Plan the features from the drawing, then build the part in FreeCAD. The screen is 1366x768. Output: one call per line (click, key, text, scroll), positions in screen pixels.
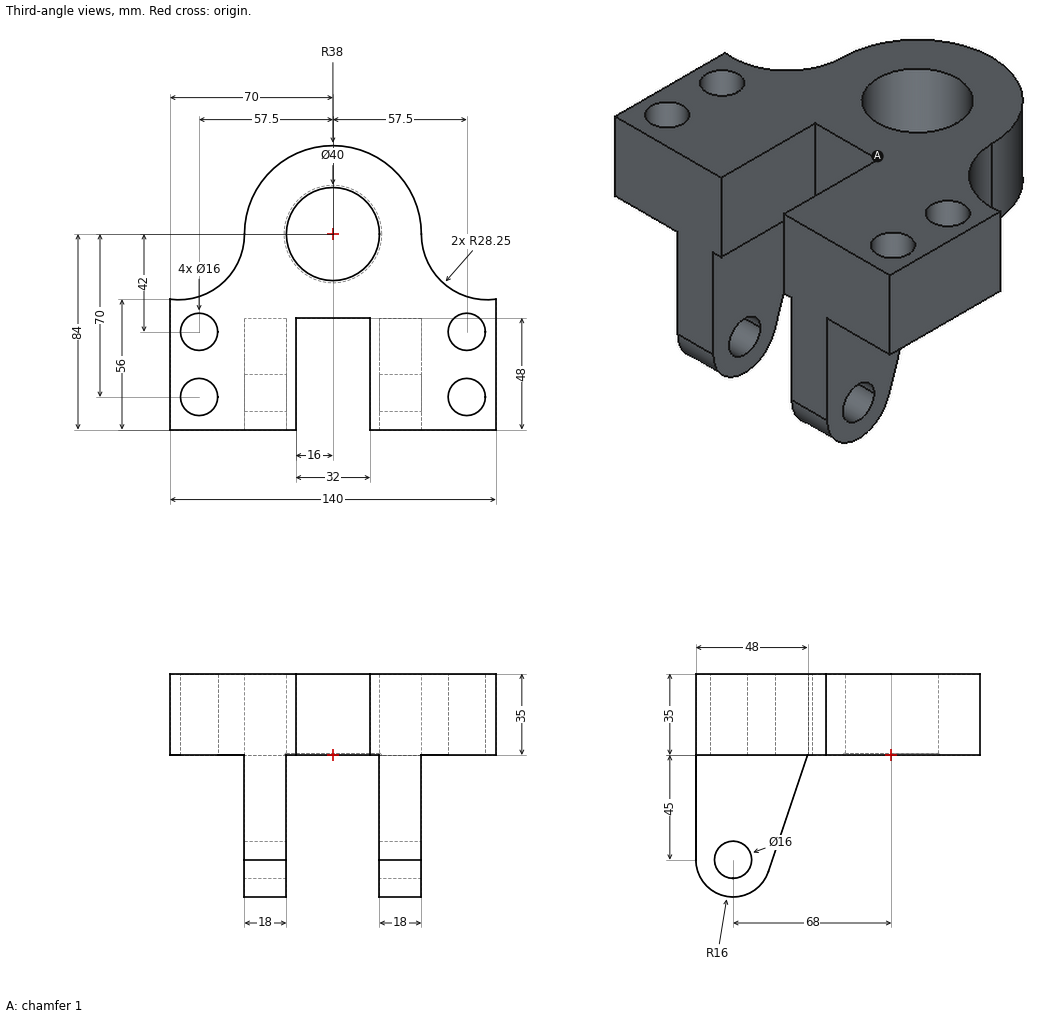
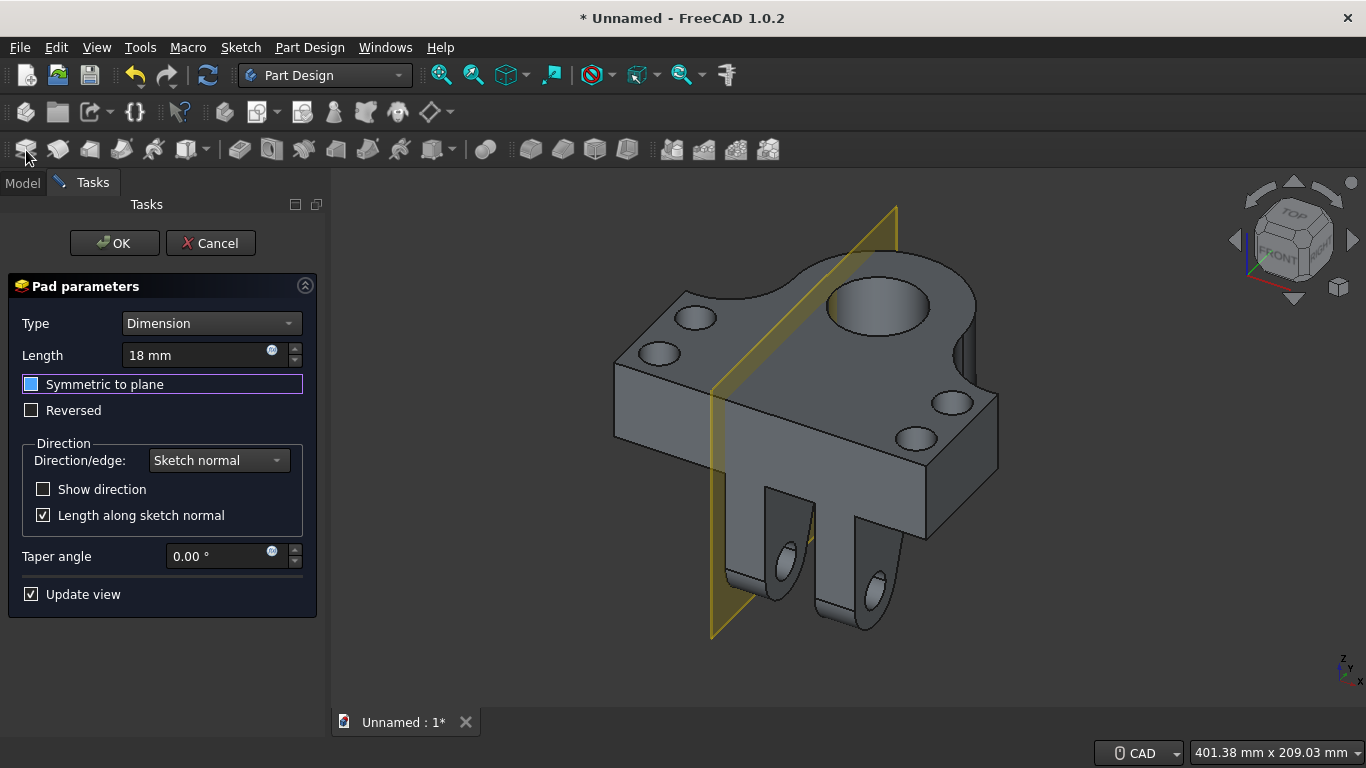
click(30, 410)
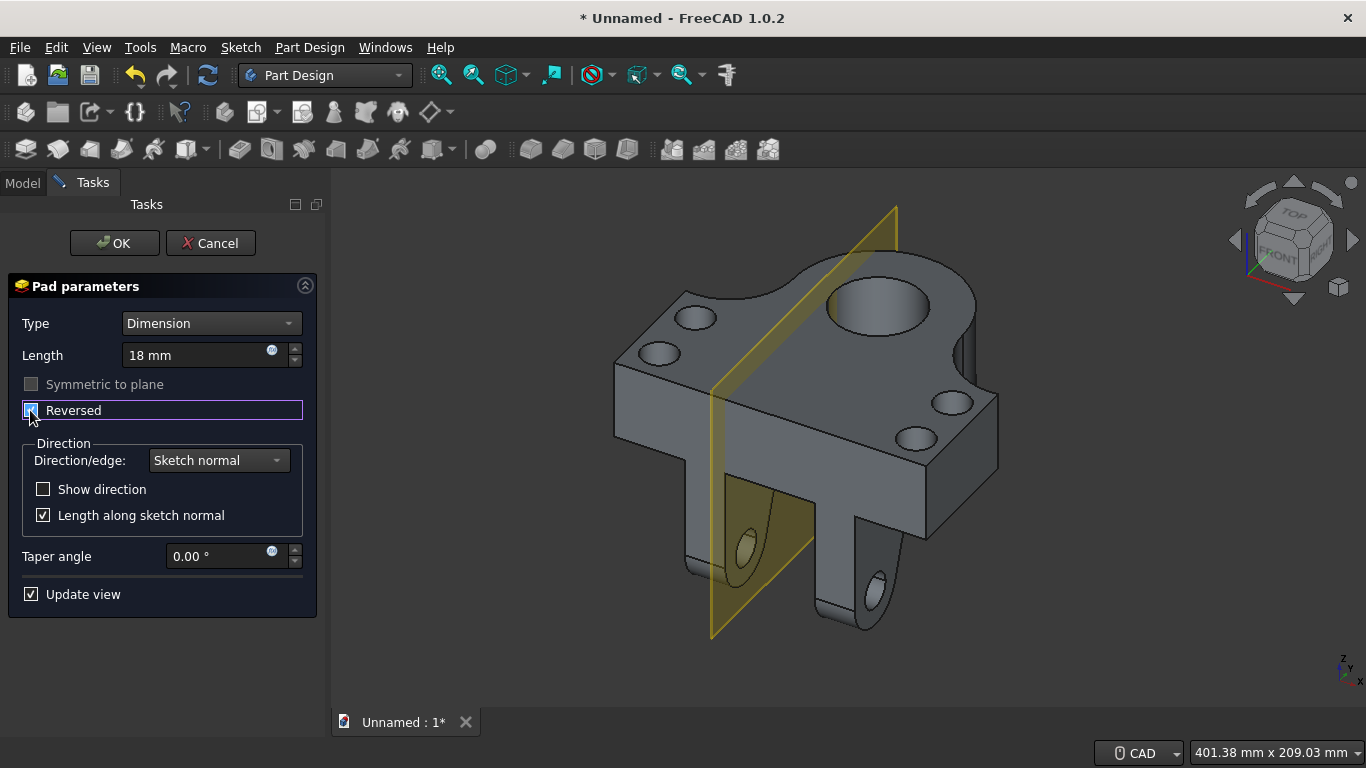
click(115, 243)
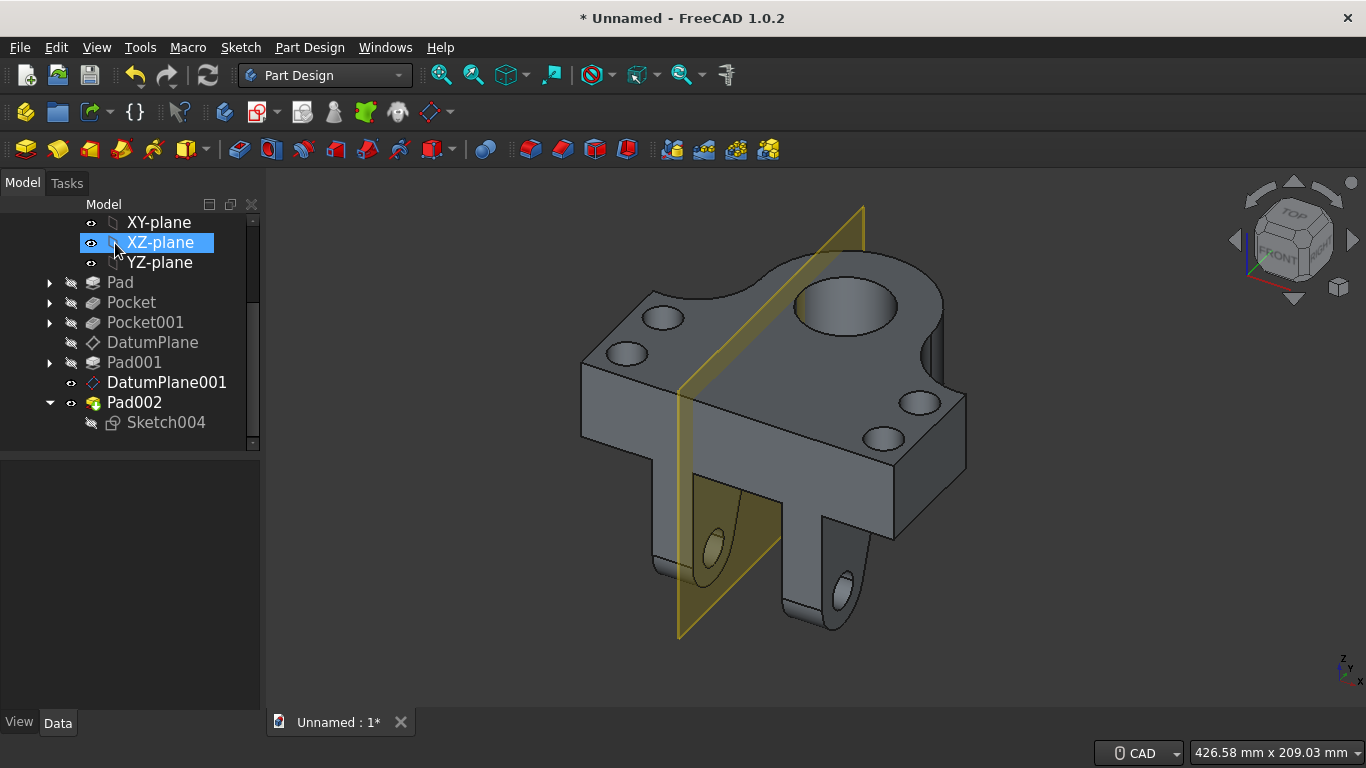
click(116, 383)
key(space)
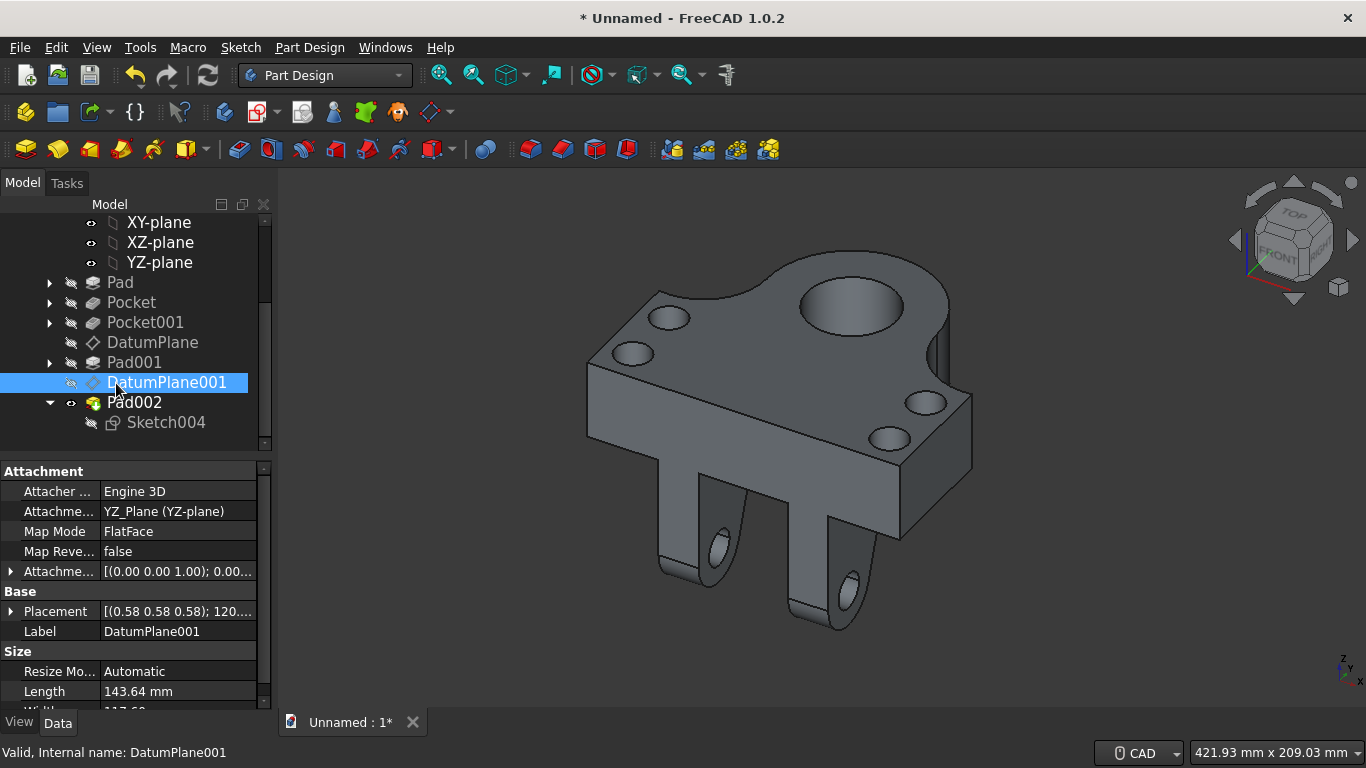
key(5)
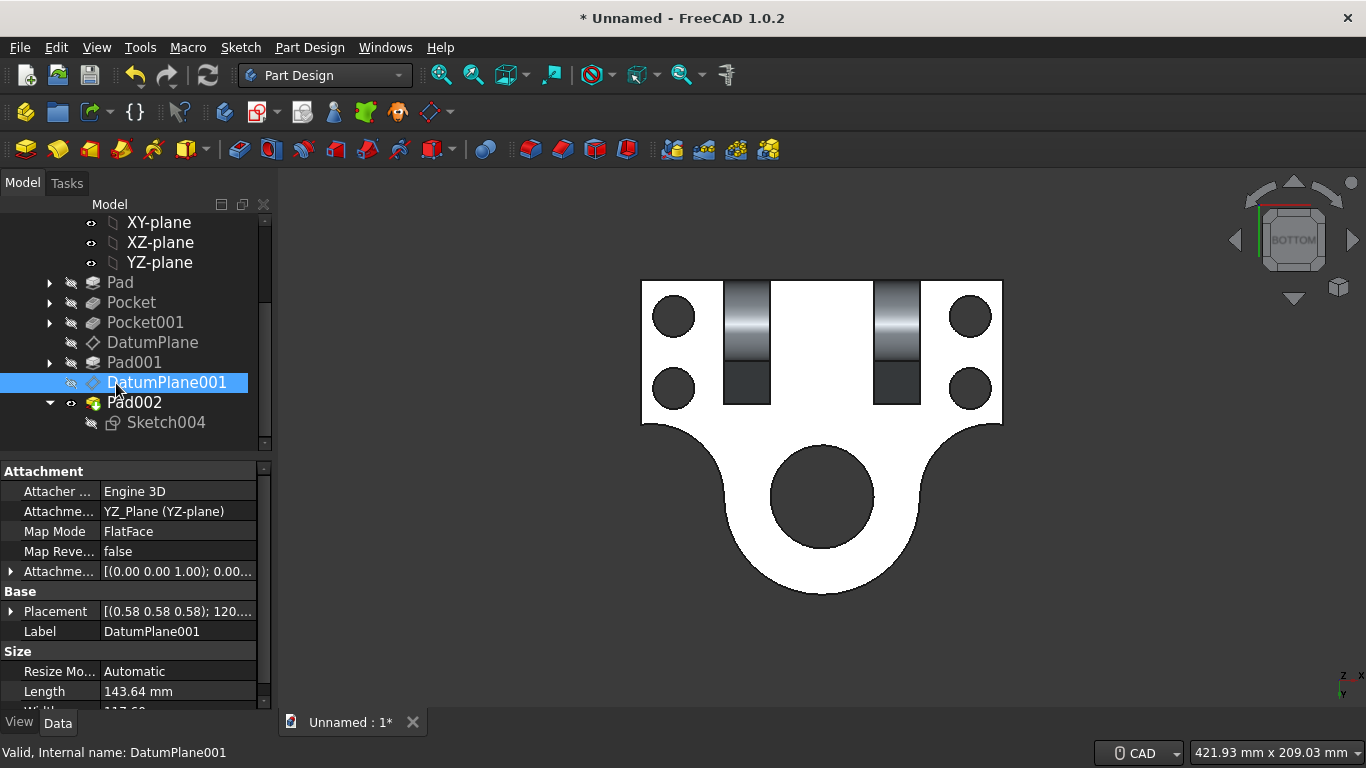
click(822, 392)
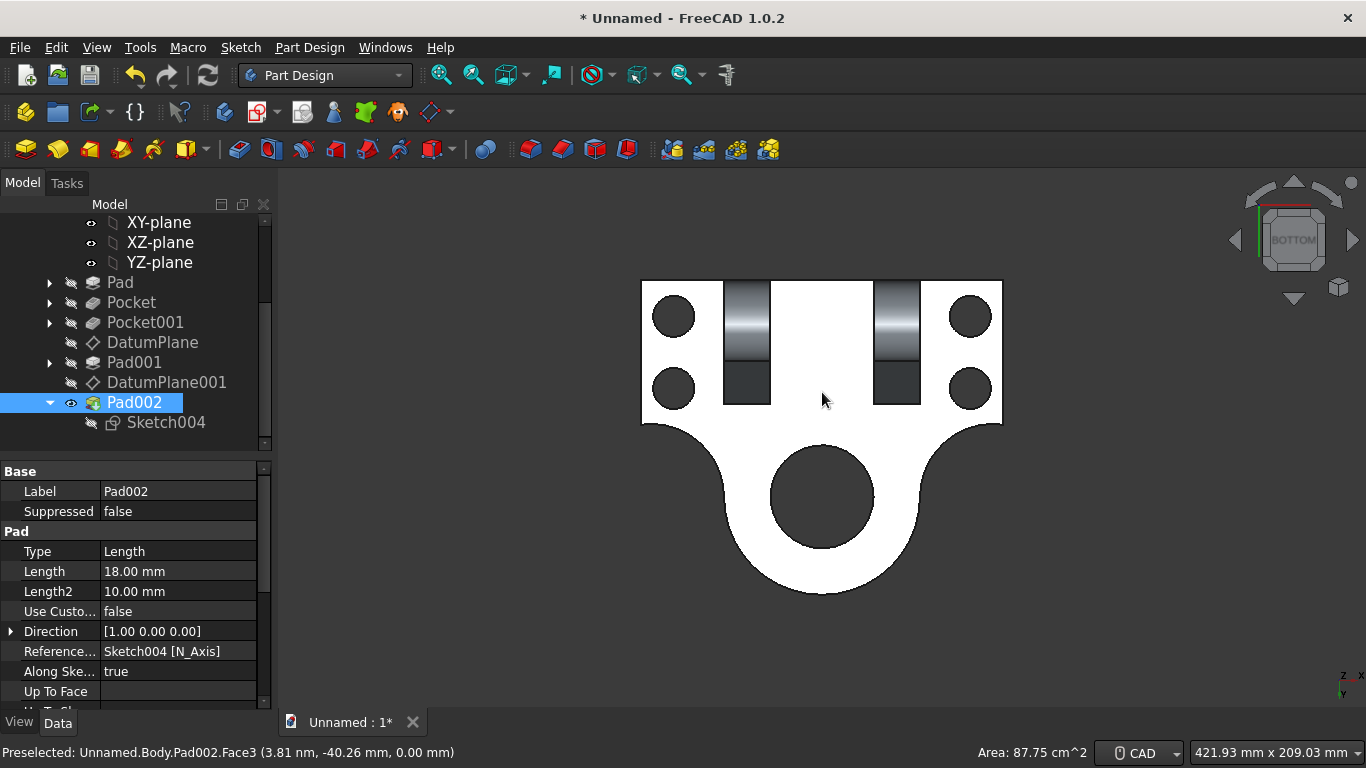
click(258, 112)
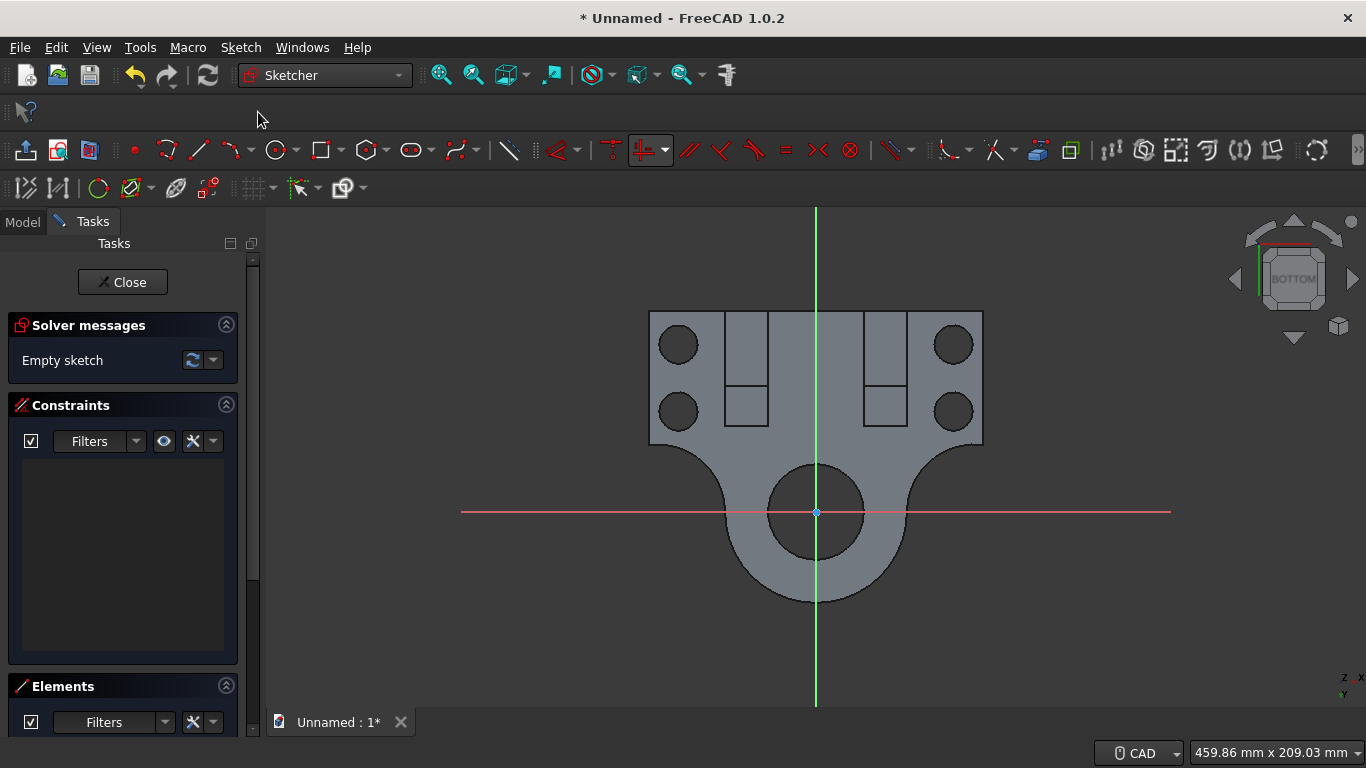
scroll(955, 319, up, 2)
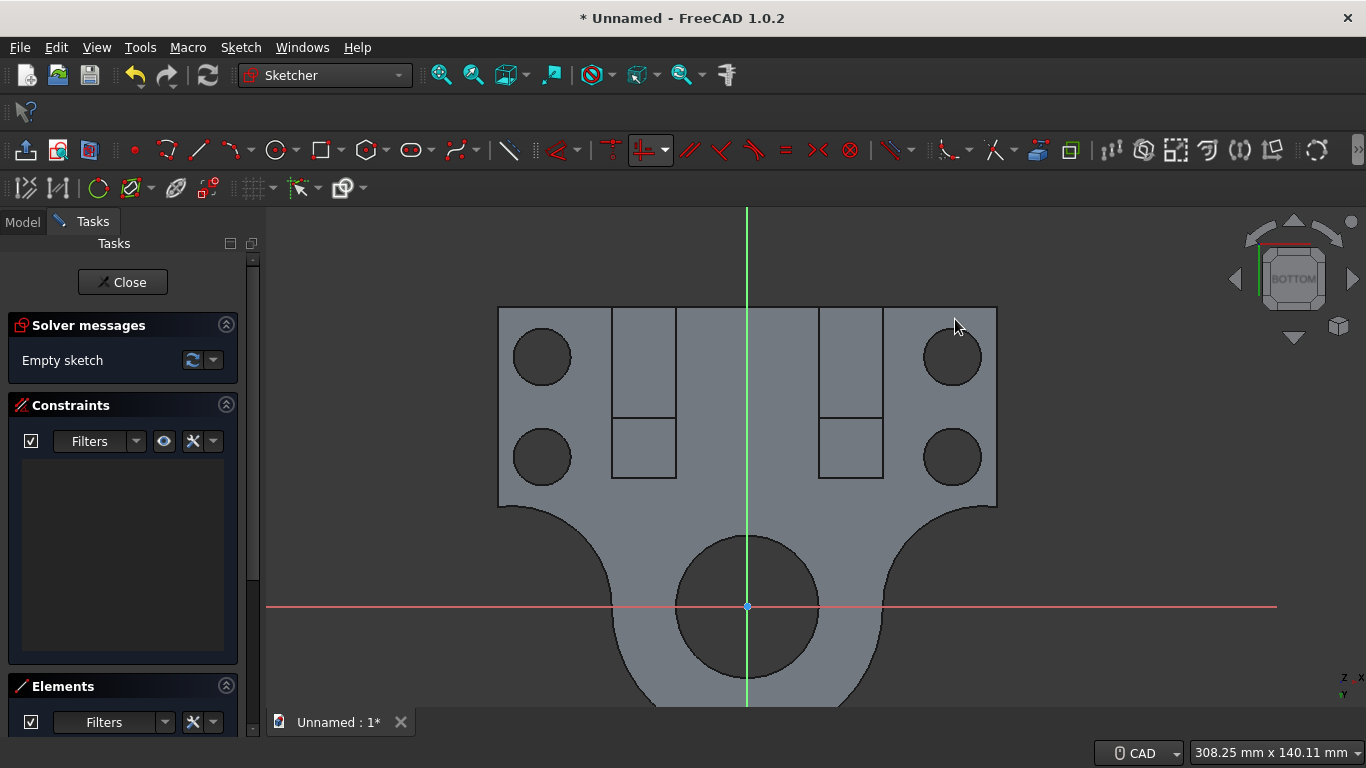
key(g)
key(r)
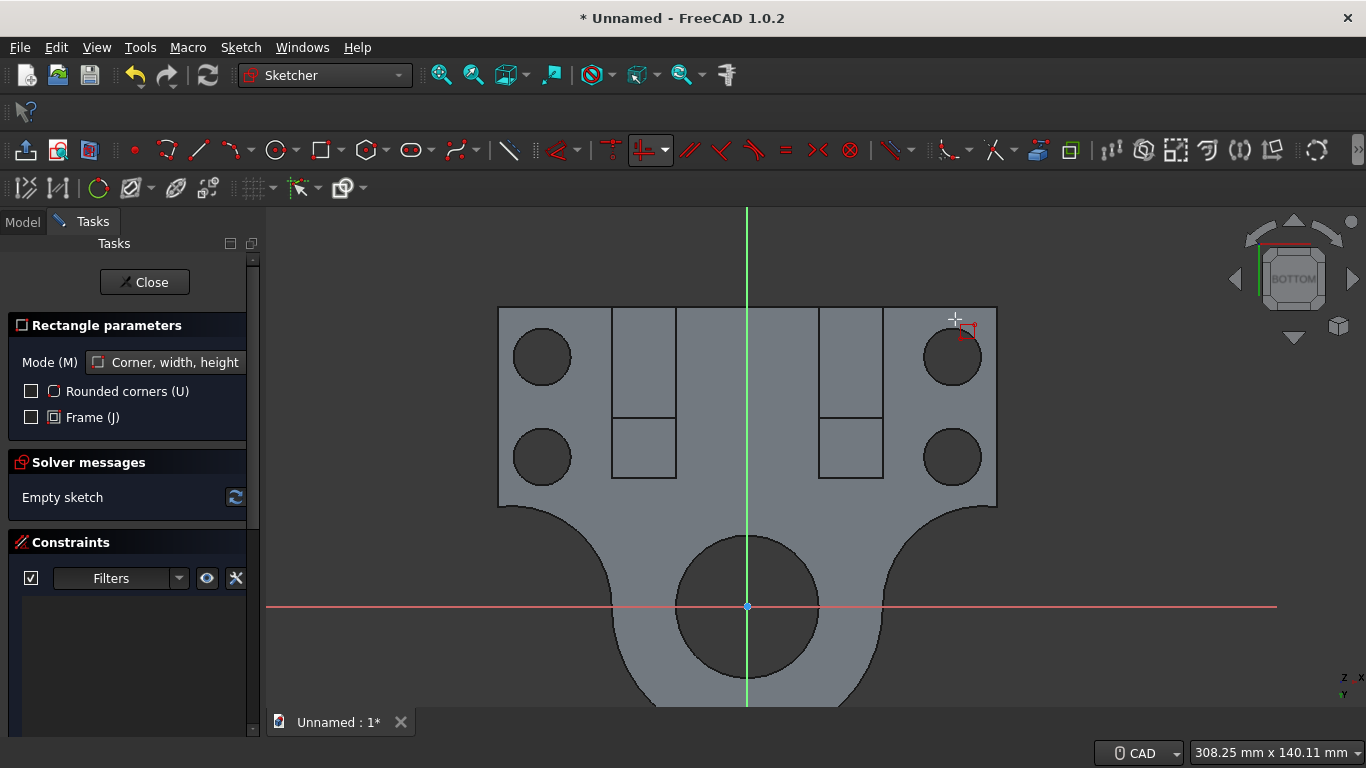
click(690, 307)
move(804, 478)